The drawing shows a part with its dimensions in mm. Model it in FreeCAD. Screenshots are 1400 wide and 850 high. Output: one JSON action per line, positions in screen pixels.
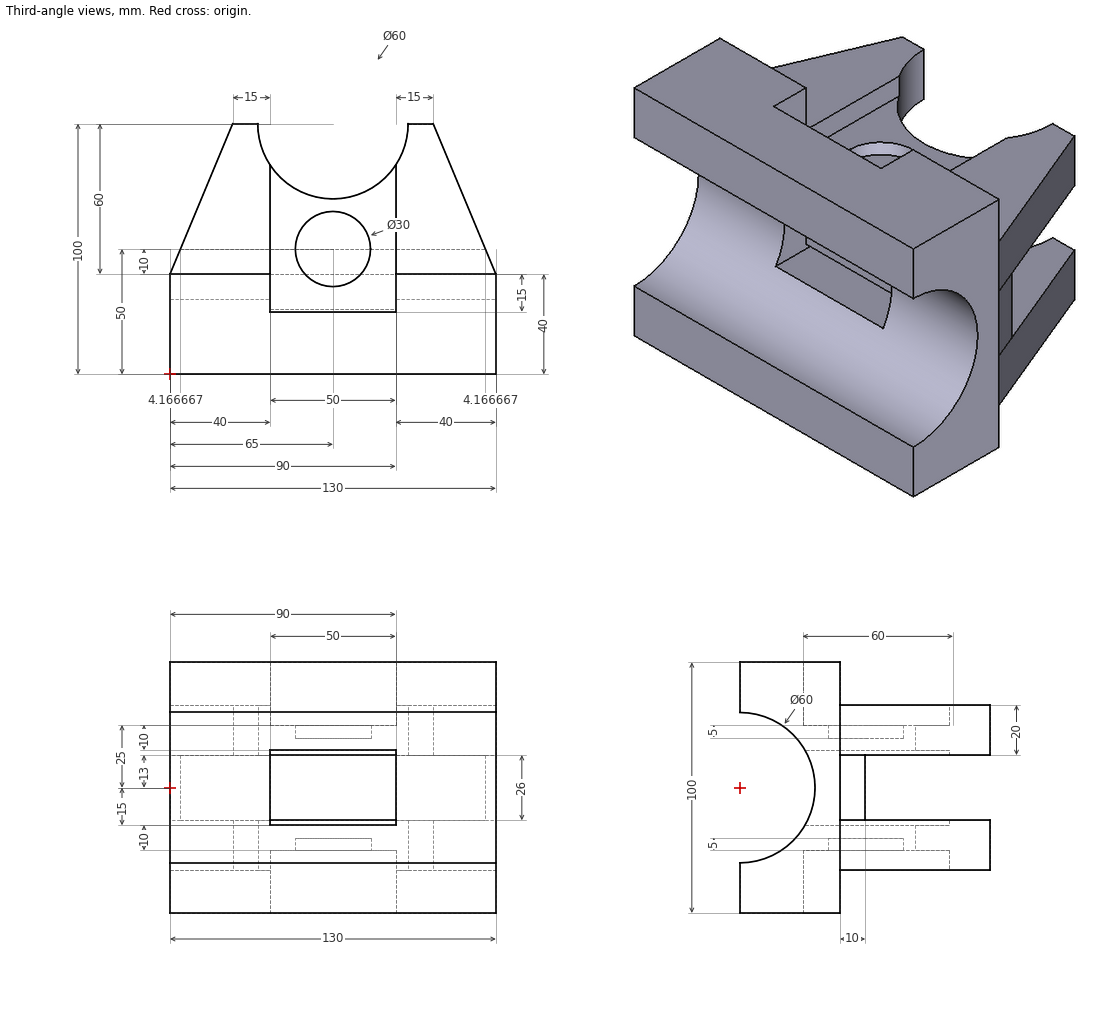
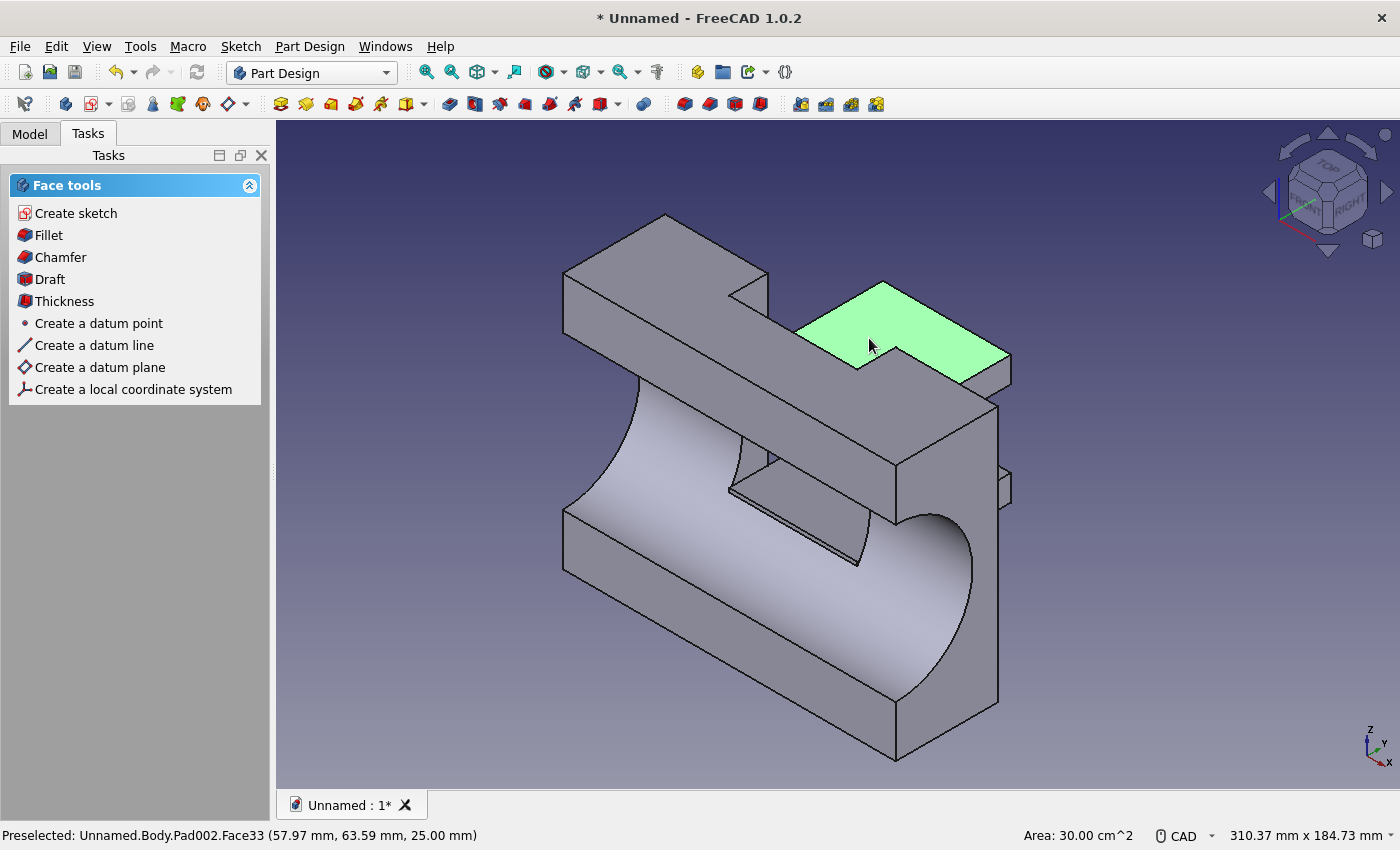
{"action": "left_click", "coordinate": [90, 104]}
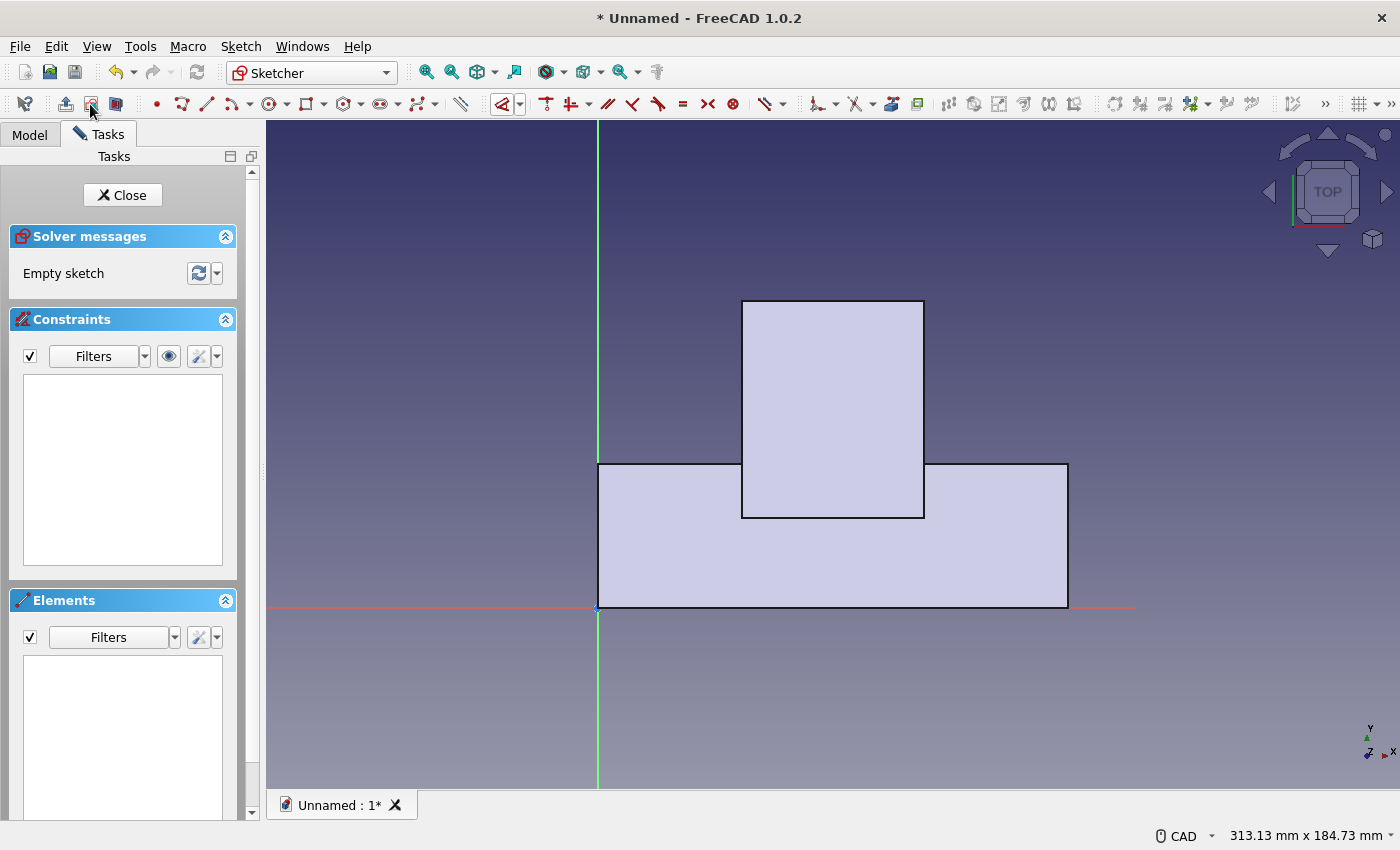
{"action": "scroll", "coordinate": [855, 418], "scroll_direction": "up", "scroll_amount": 7}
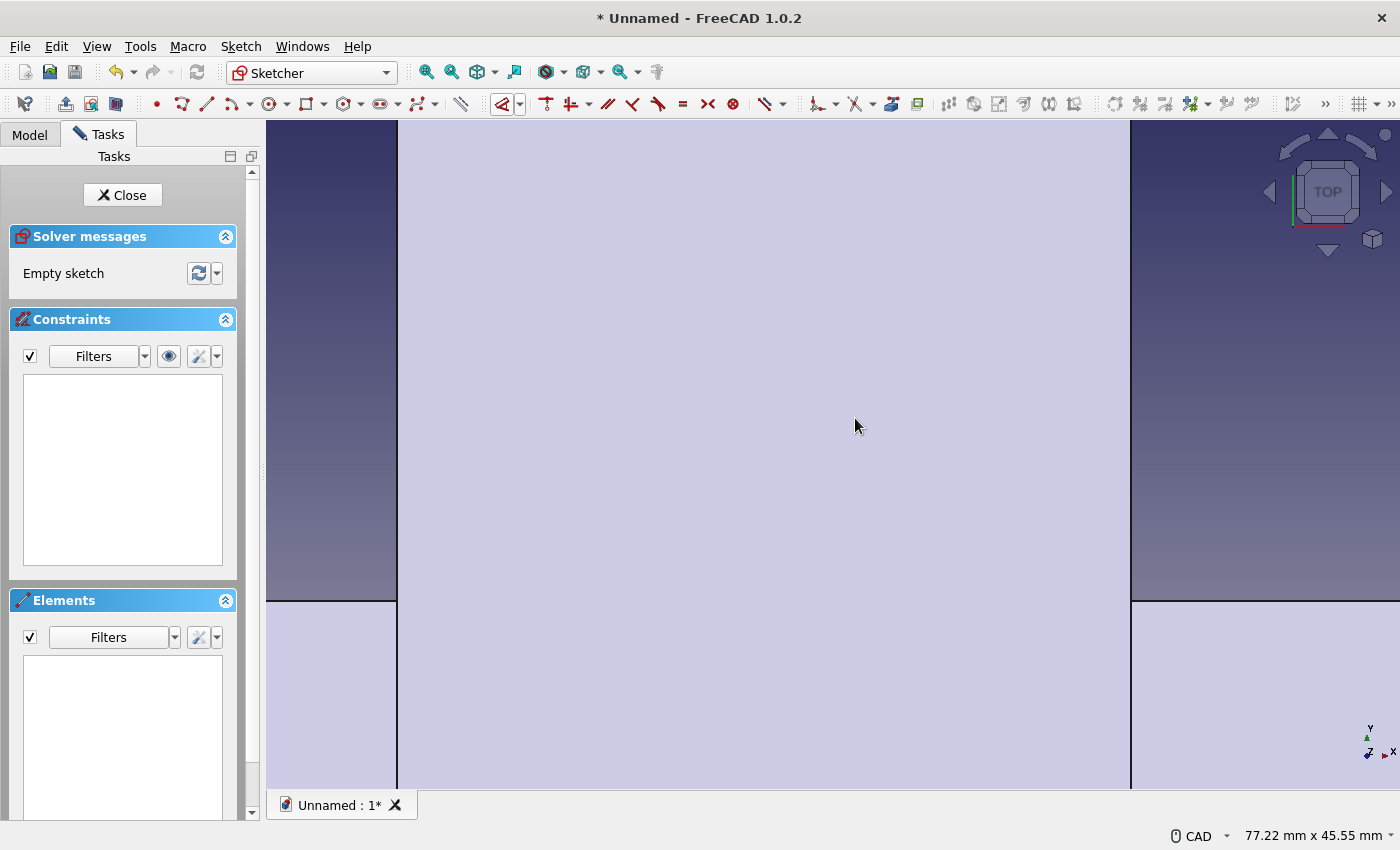
{"action": "left_click", "coordinate": [268, 104]}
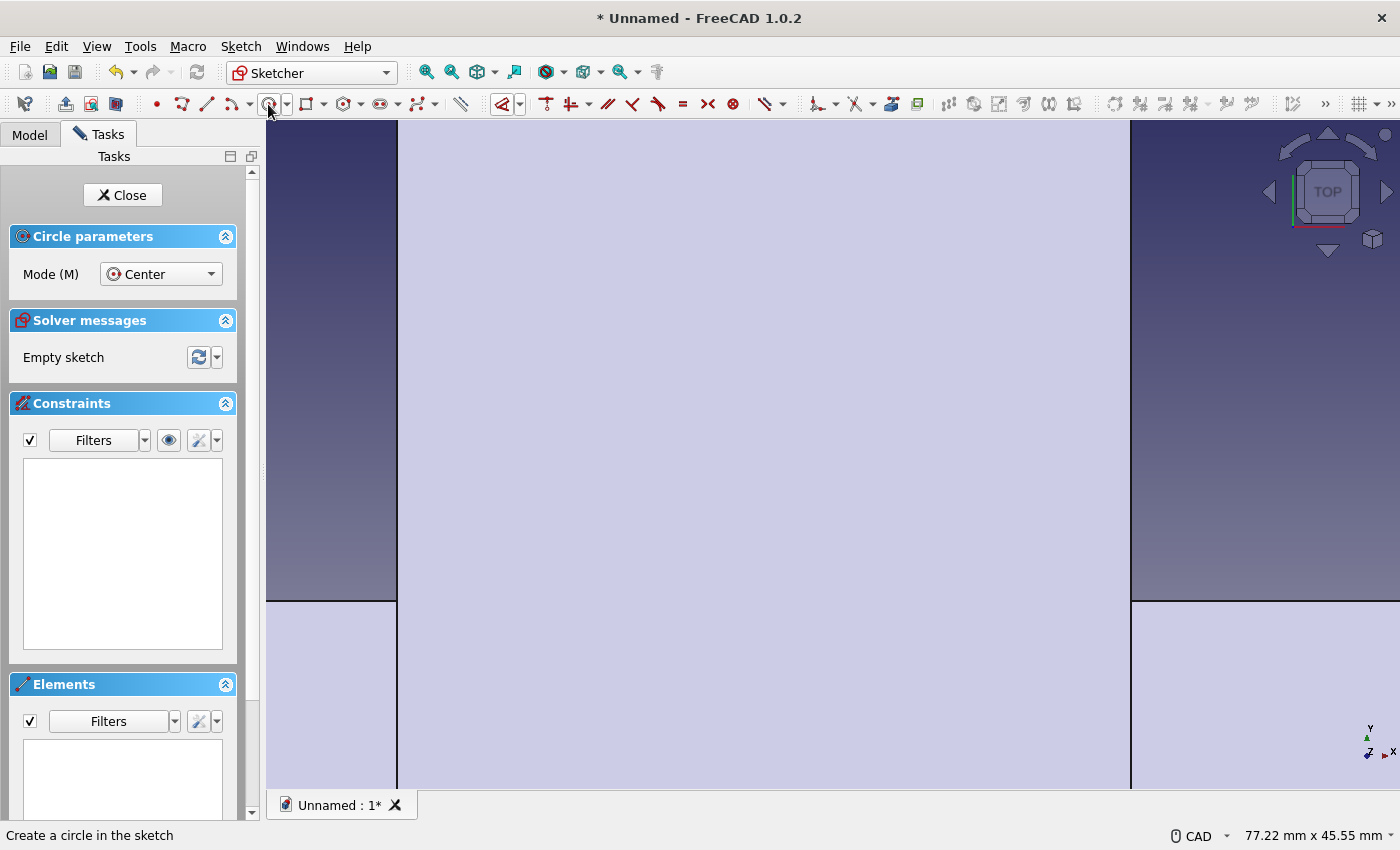
{"action": "left_click", "coordinate": [764, 455]}
{"action": "mouse_move", "coordinate": [920, 299]}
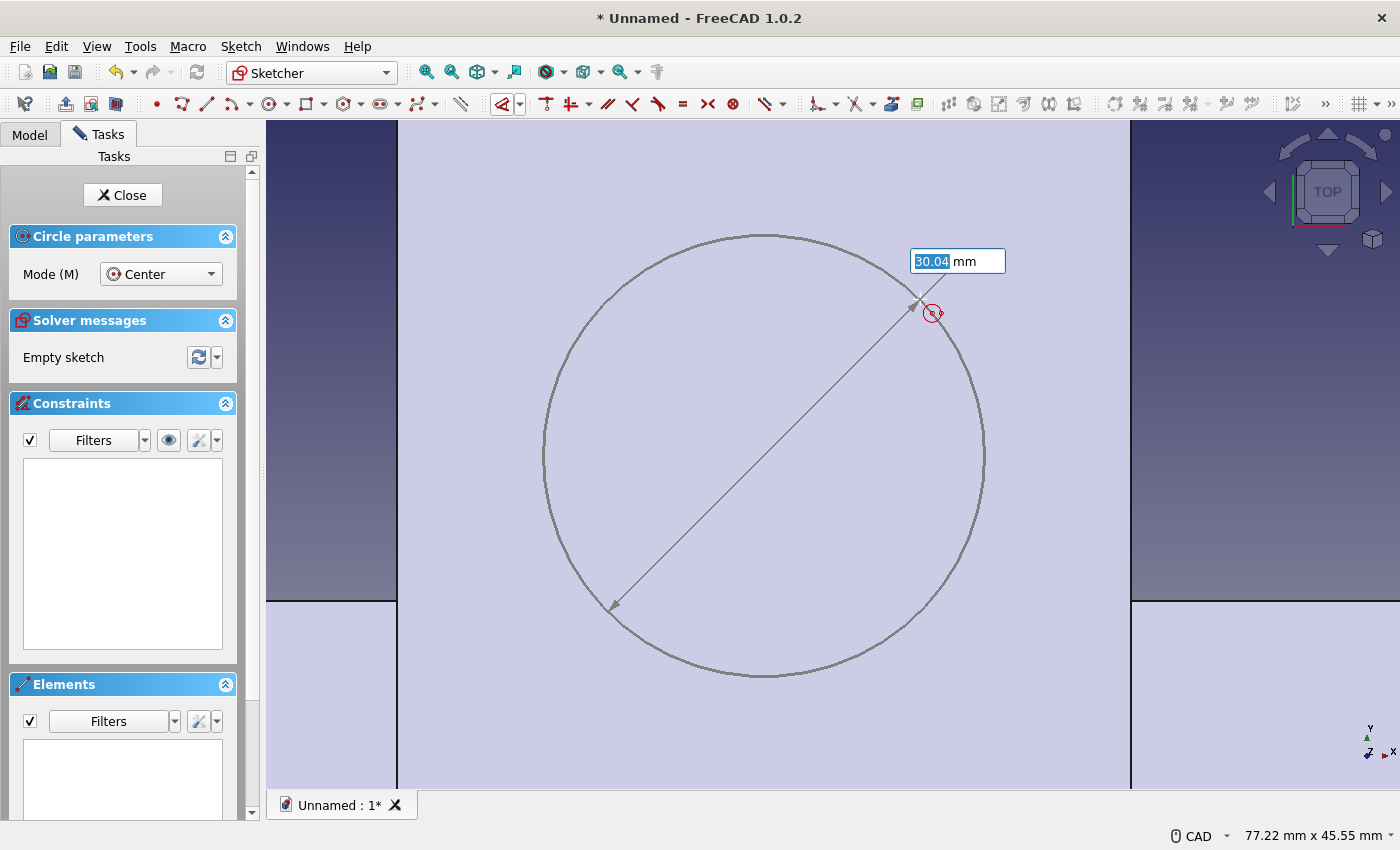
{"action": "type", "text": "30"}
{"action": "key", "text": "Return"}
{"action": "key", "text": "Escape"}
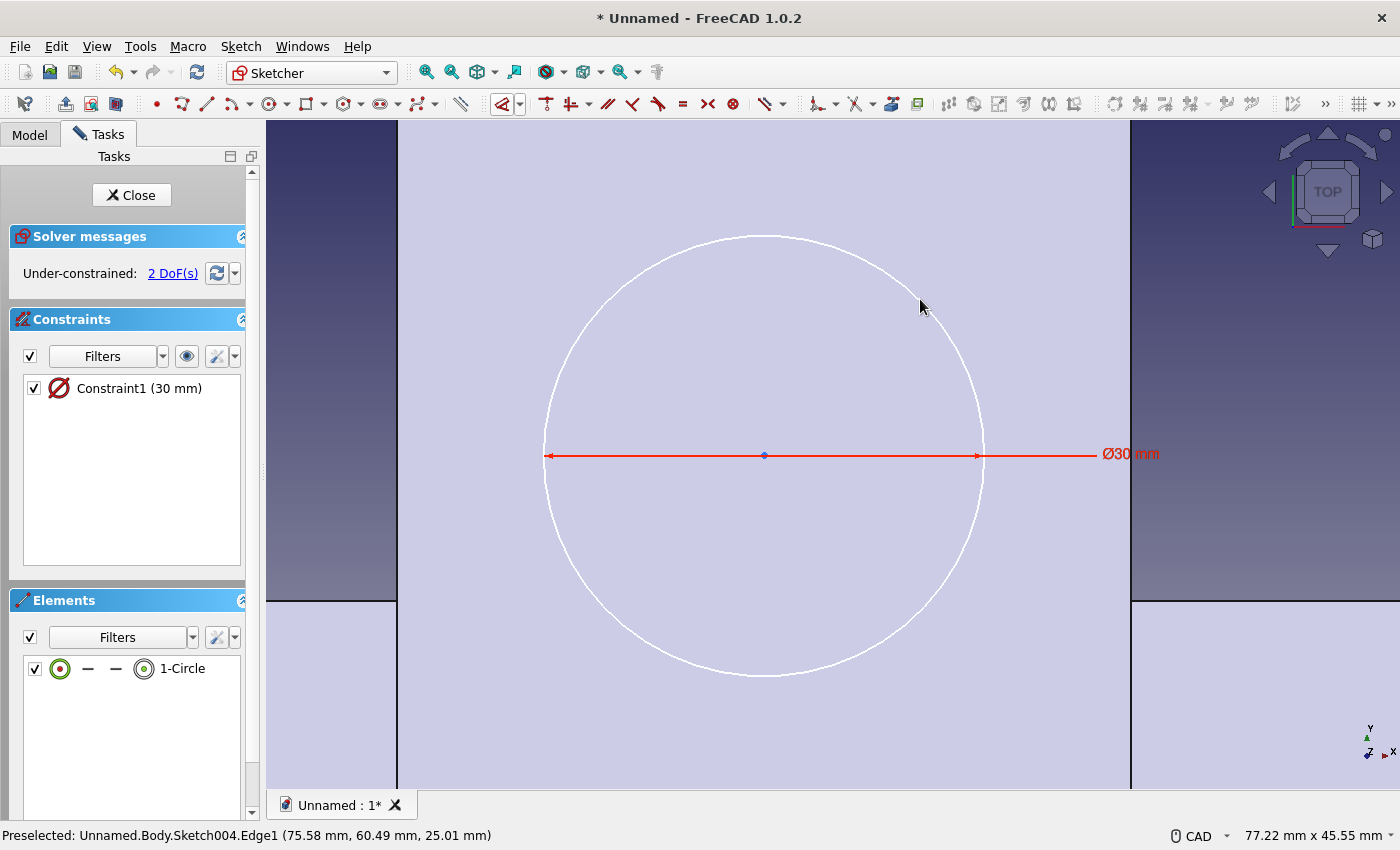
{"action": "left_click", "coordinate": [764, 456]}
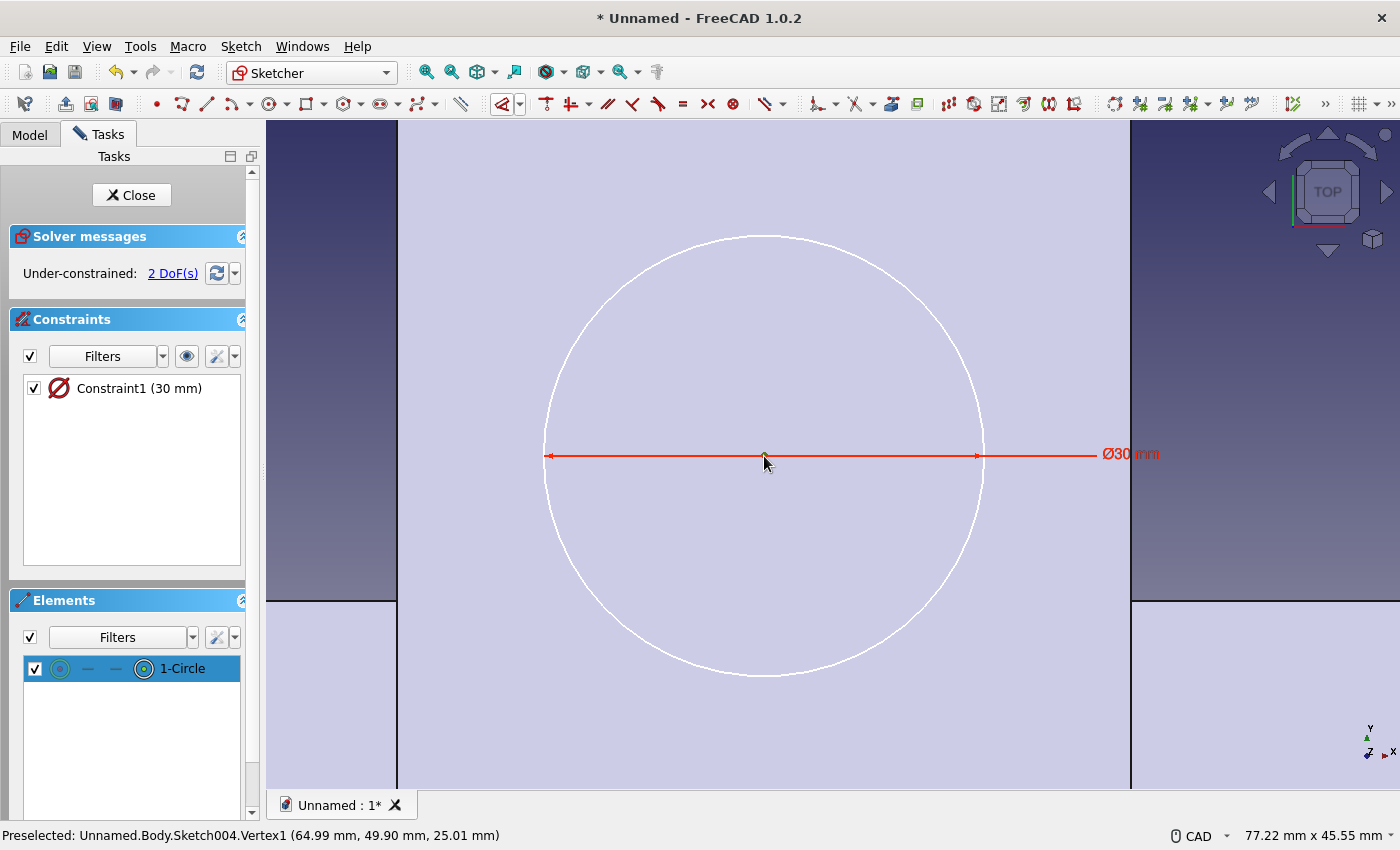
{"action": "key", "text": "l"}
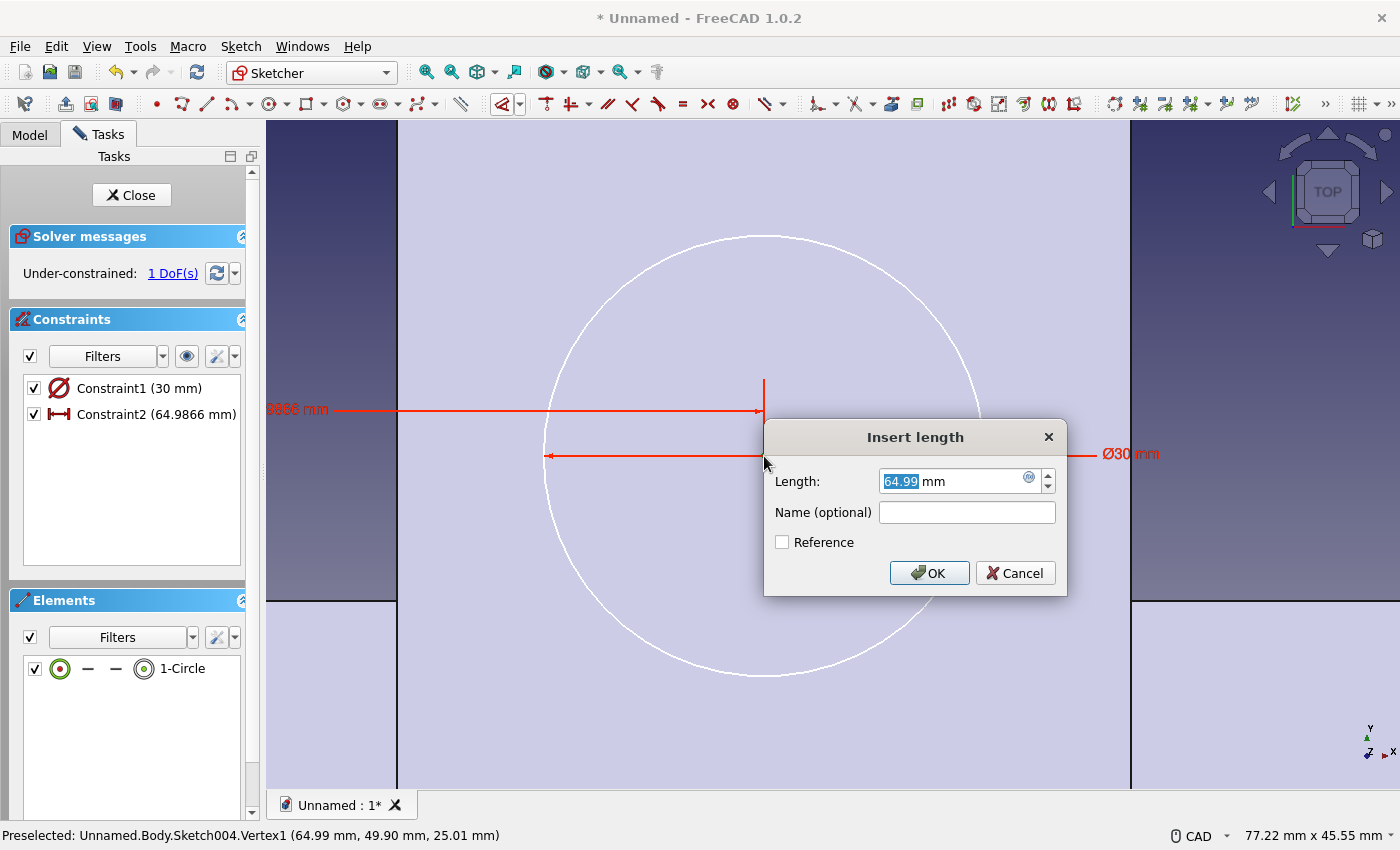
{"action": "type", "text": "65"}
{"action": "key", "text": "Return"}